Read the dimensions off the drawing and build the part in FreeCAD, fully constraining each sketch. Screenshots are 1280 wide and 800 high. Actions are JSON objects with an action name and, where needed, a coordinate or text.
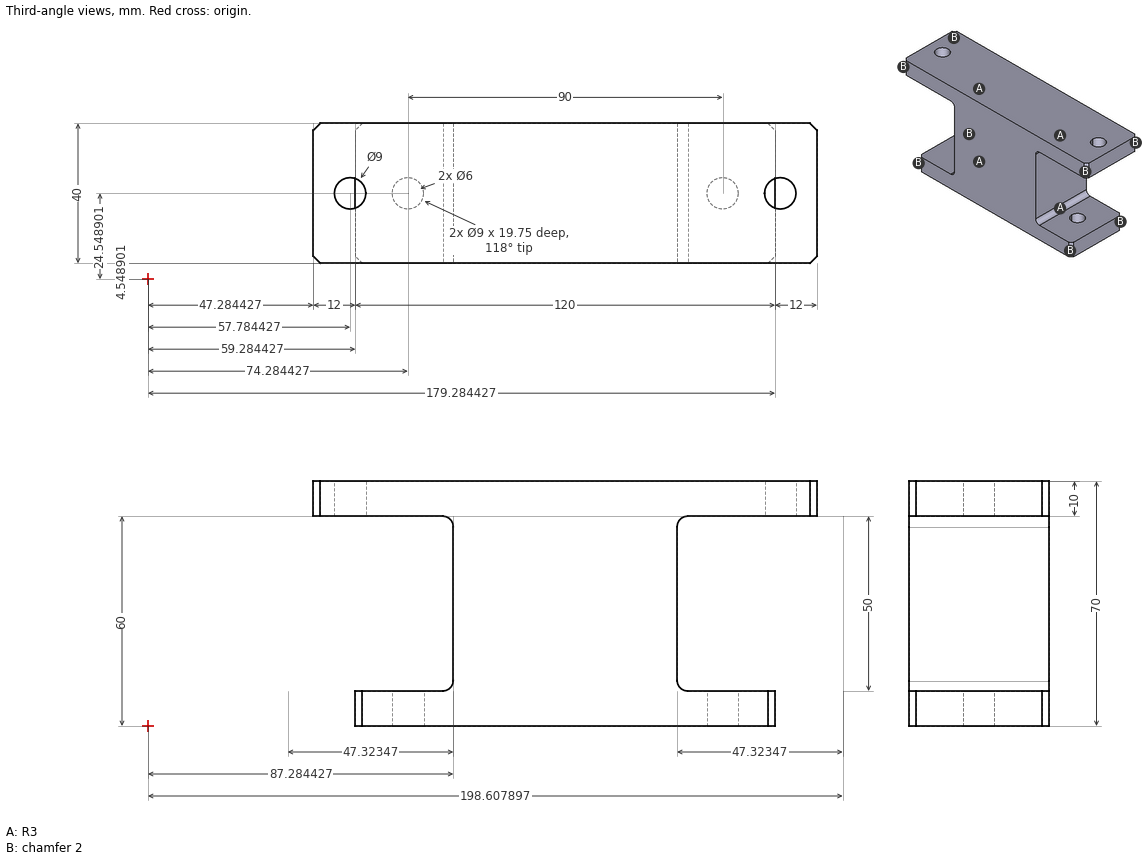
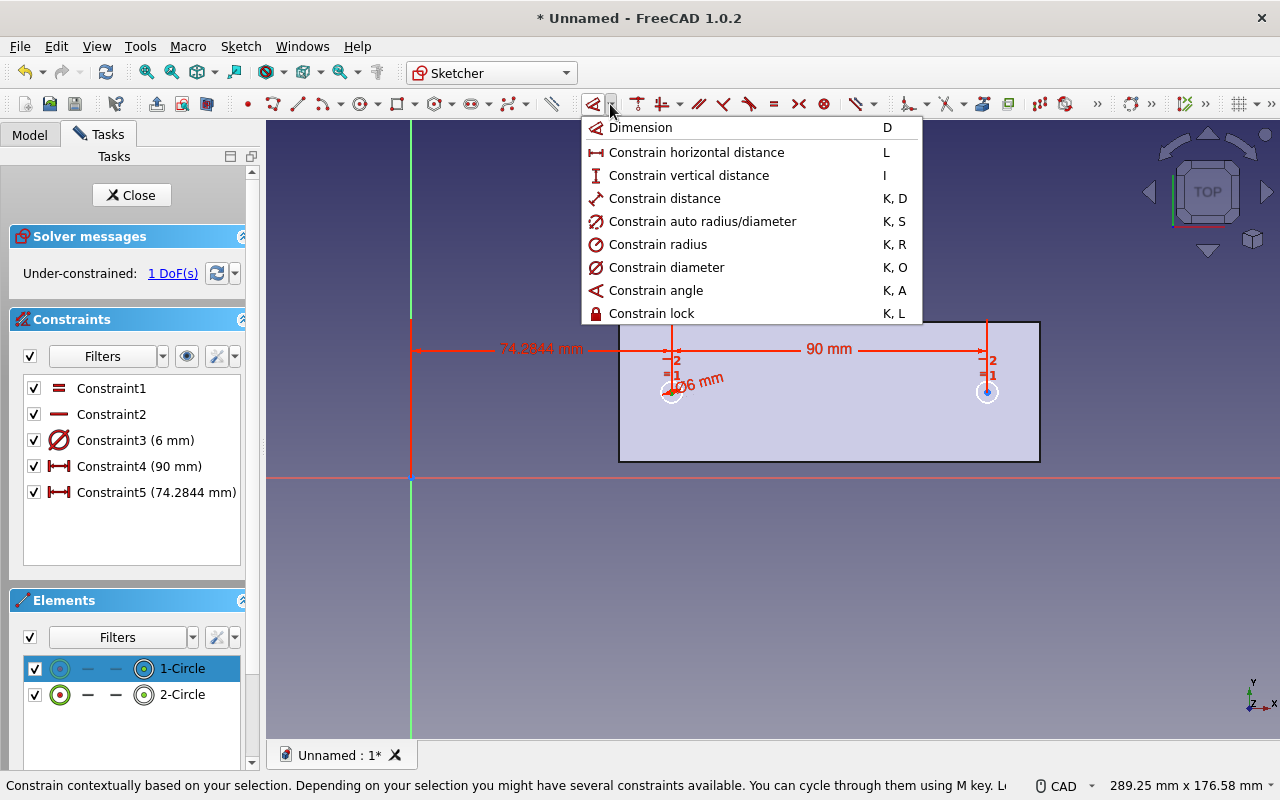
{"action": "left_click", "coordinate": [752, 176]}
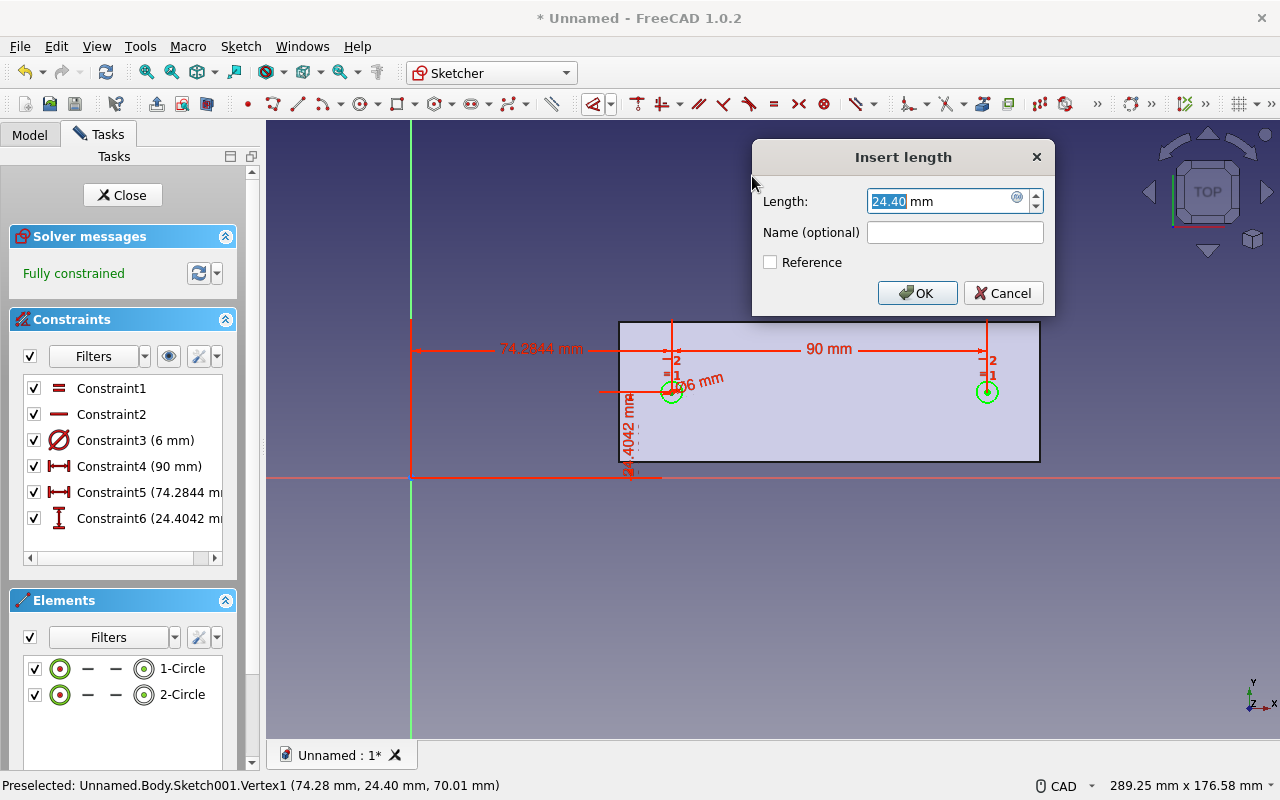
{"action": "type", "text": "24.548901"}
{"action": "key", "text": "Return"}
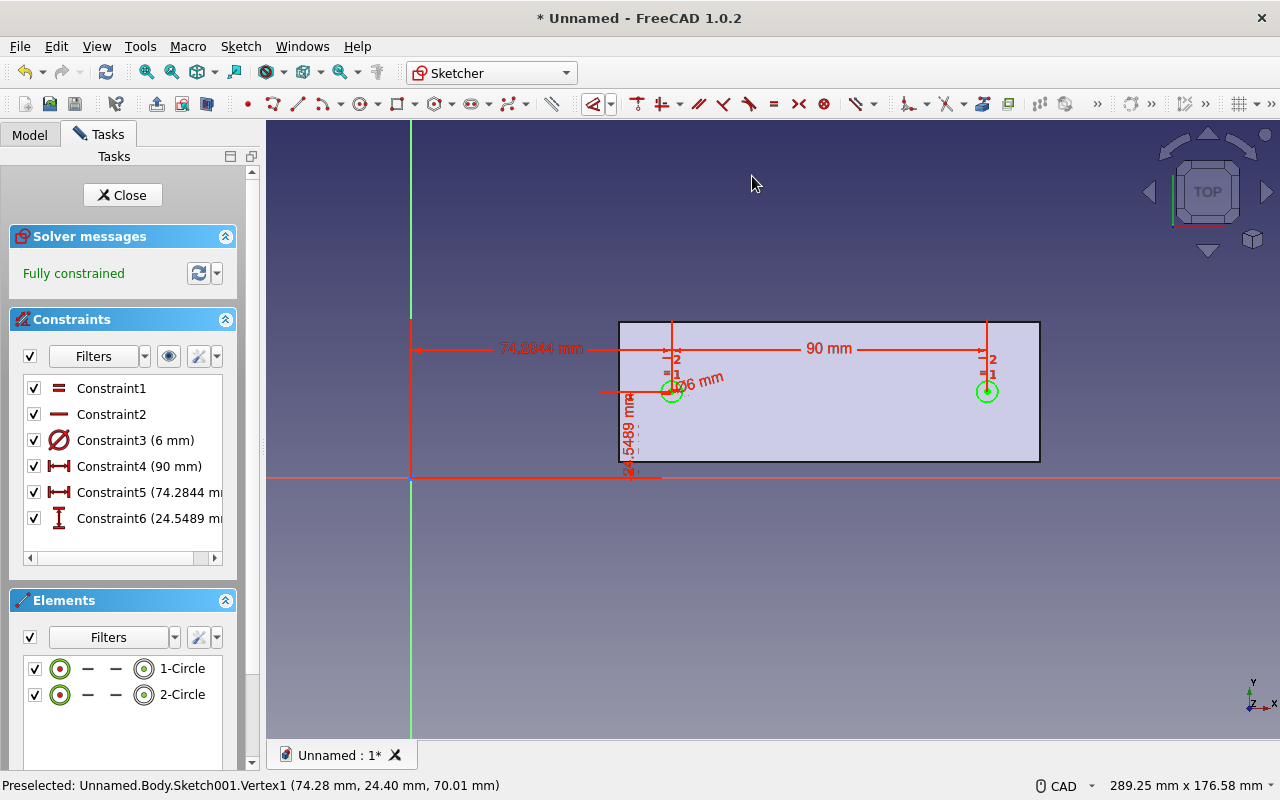
{"action": "left_click", "coordinate": [123, 195]}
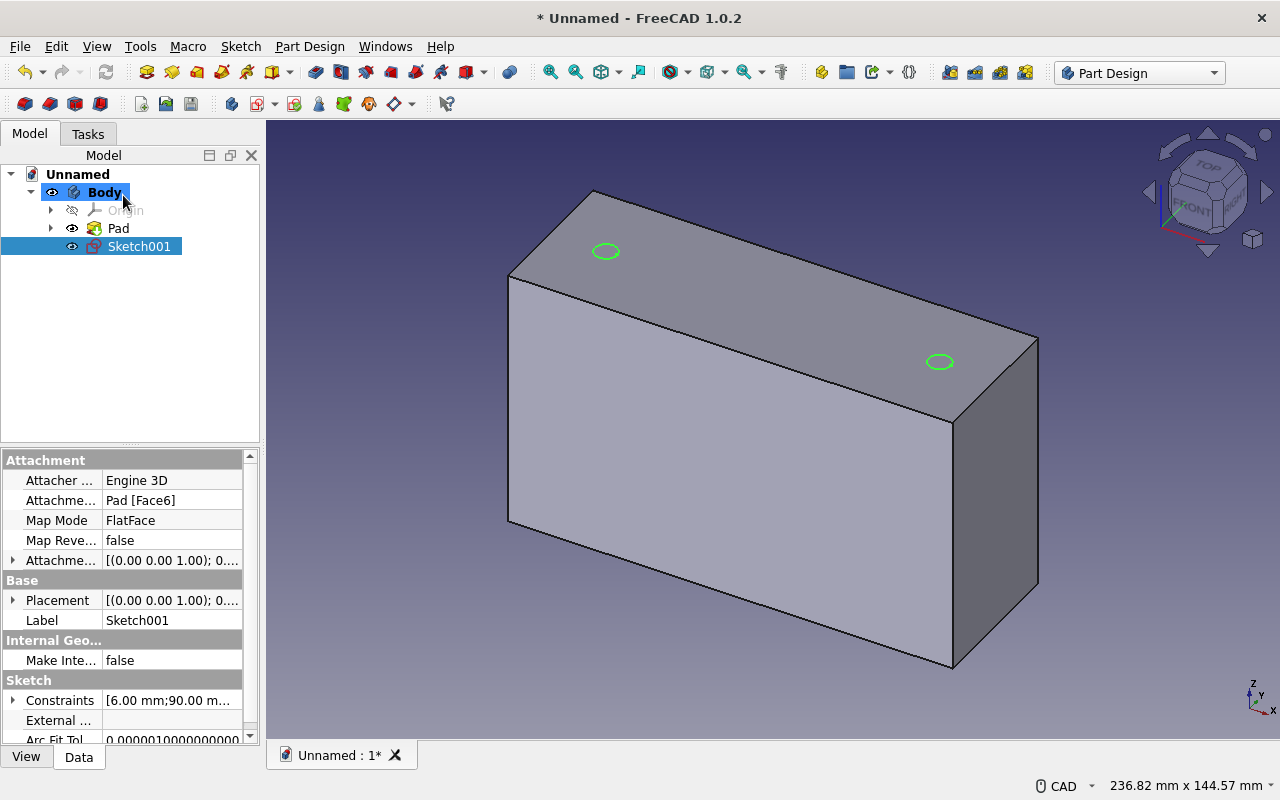
{"action": "left_click", "coordinate": [316, 72]}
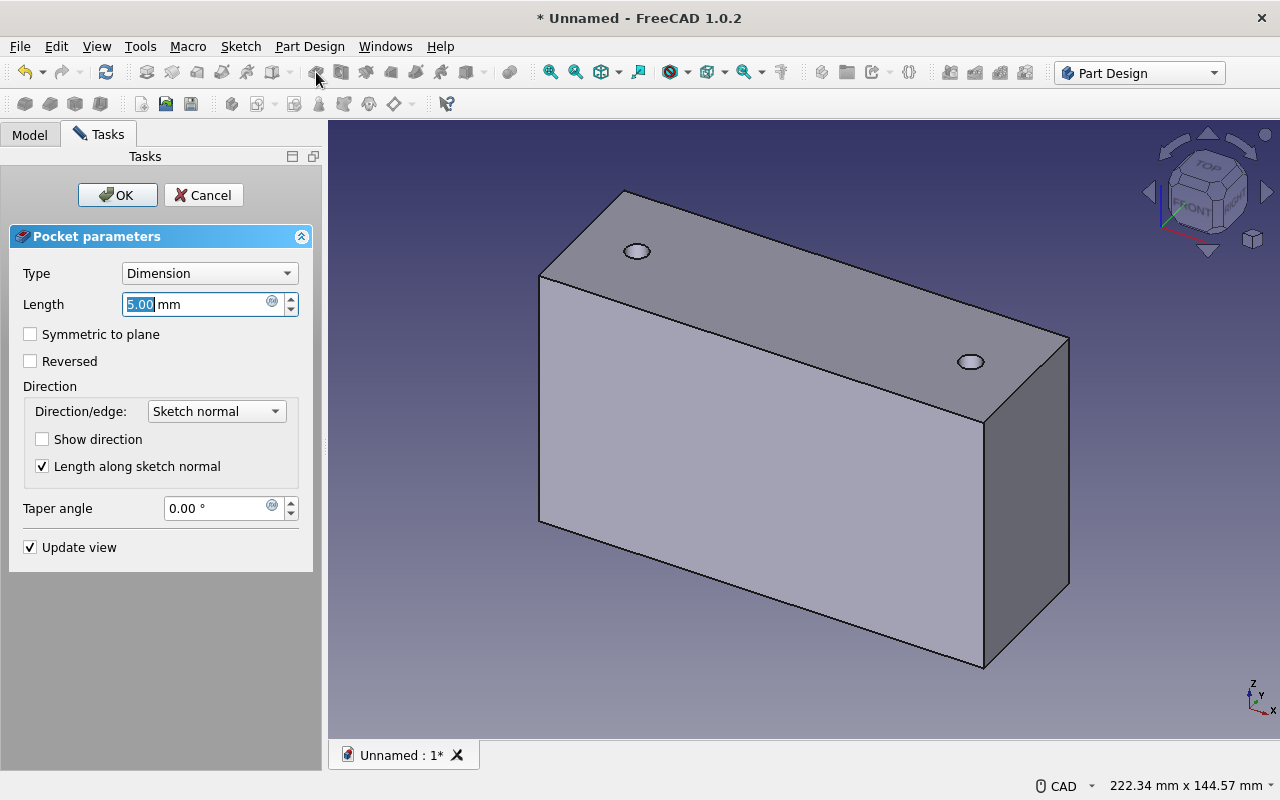
{"action": "left_click", "coordinate": [210, 274]}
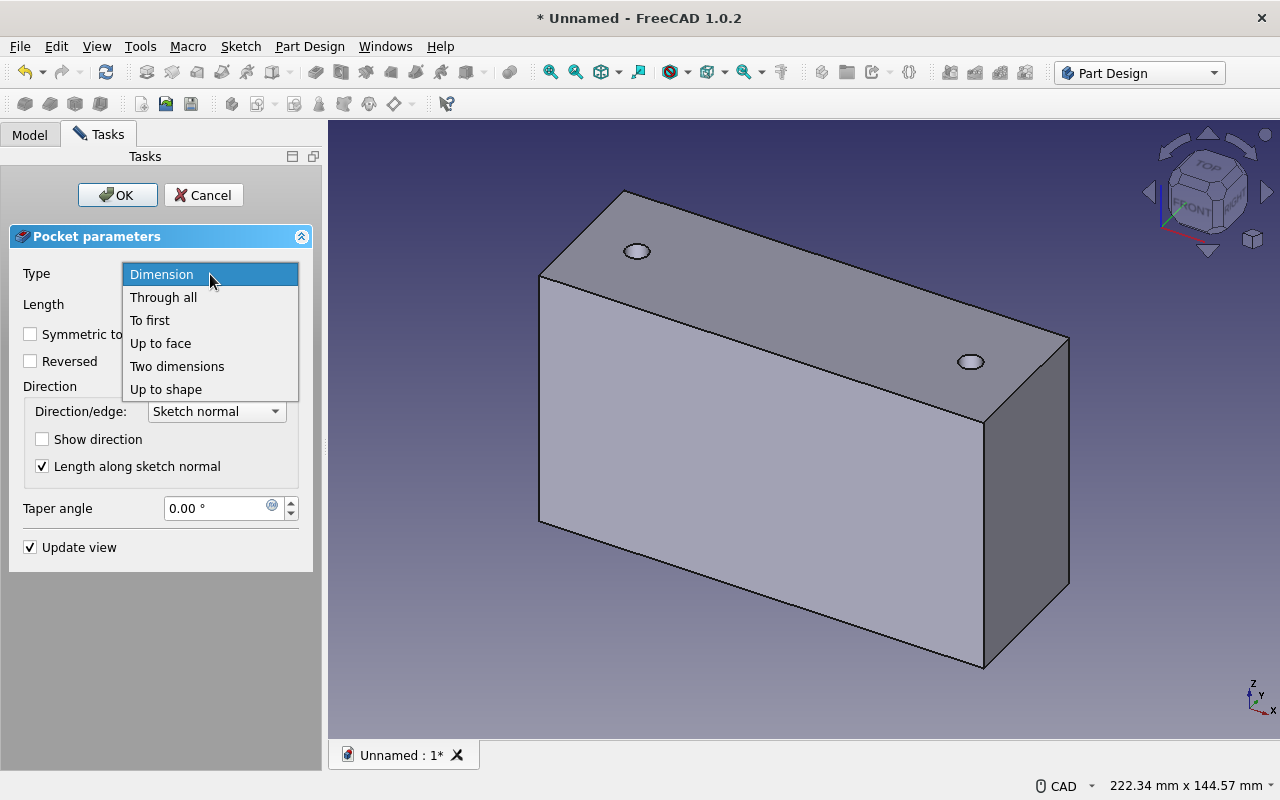
{"action": "left_click", "coordinate": [208, 298]}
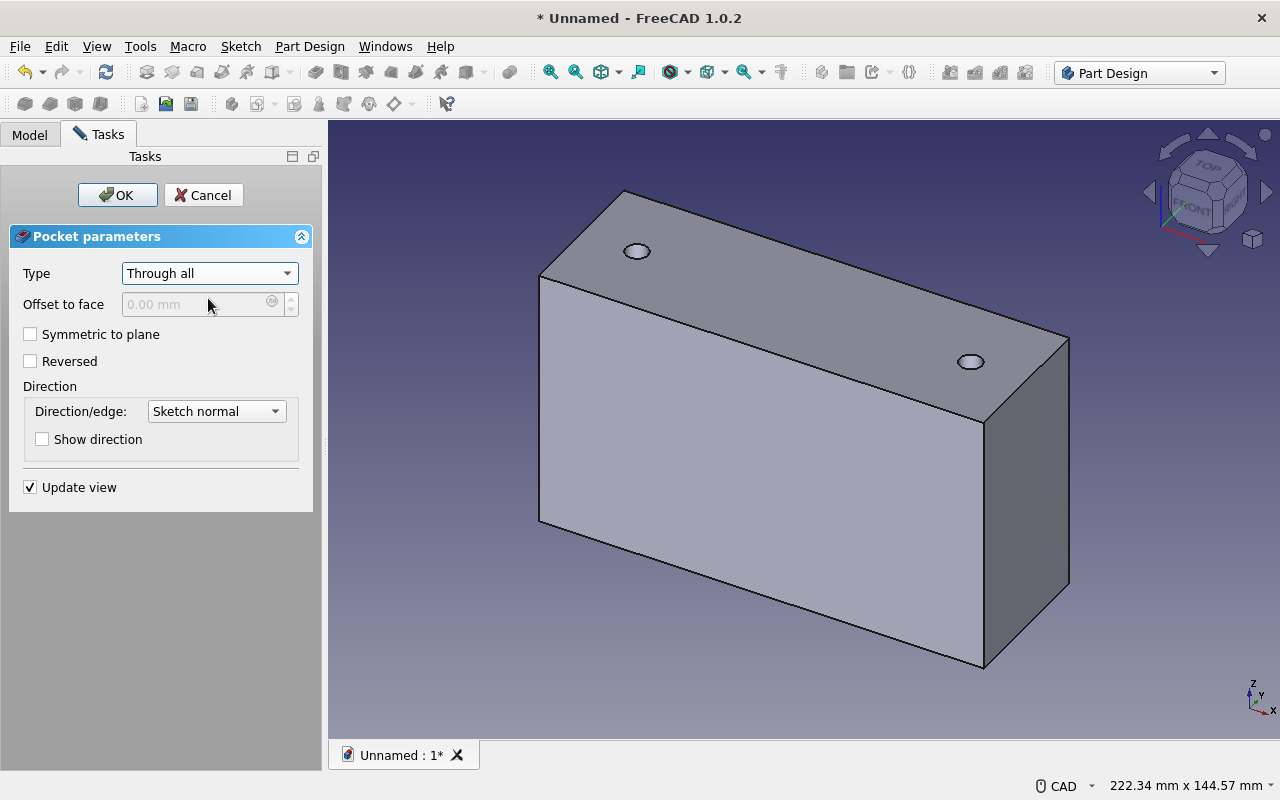
{"action": "left_click", "coordinate": [118, 195]}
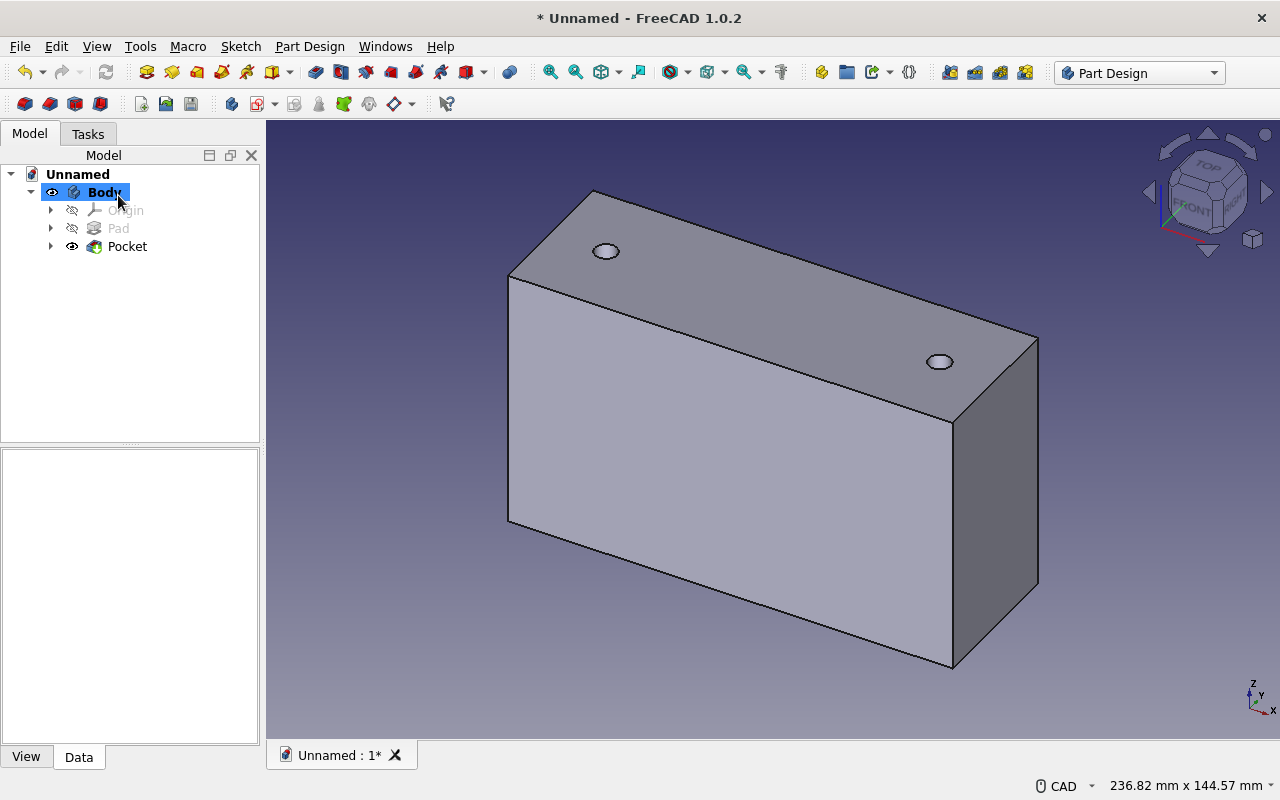
{"action": "key", "text": "4"}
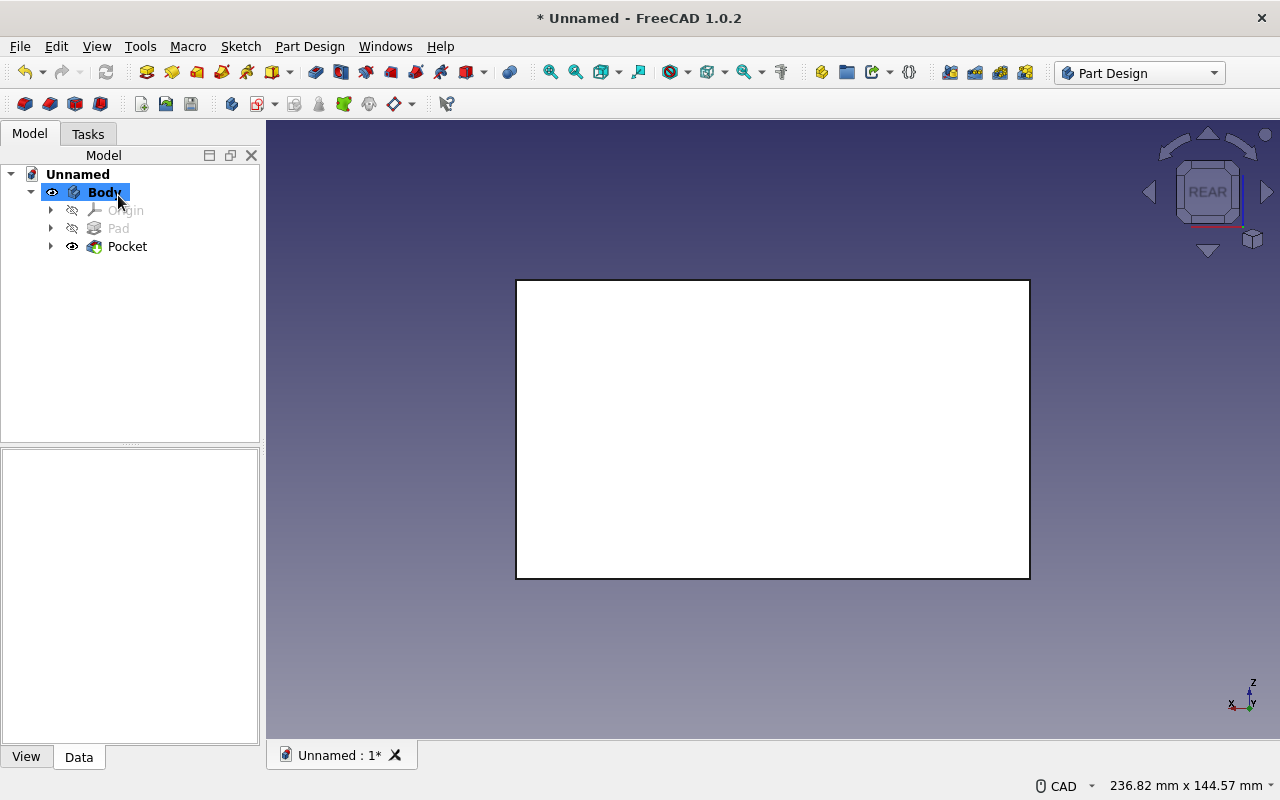
{"action": "left_click", "coordinate": [700, 428]}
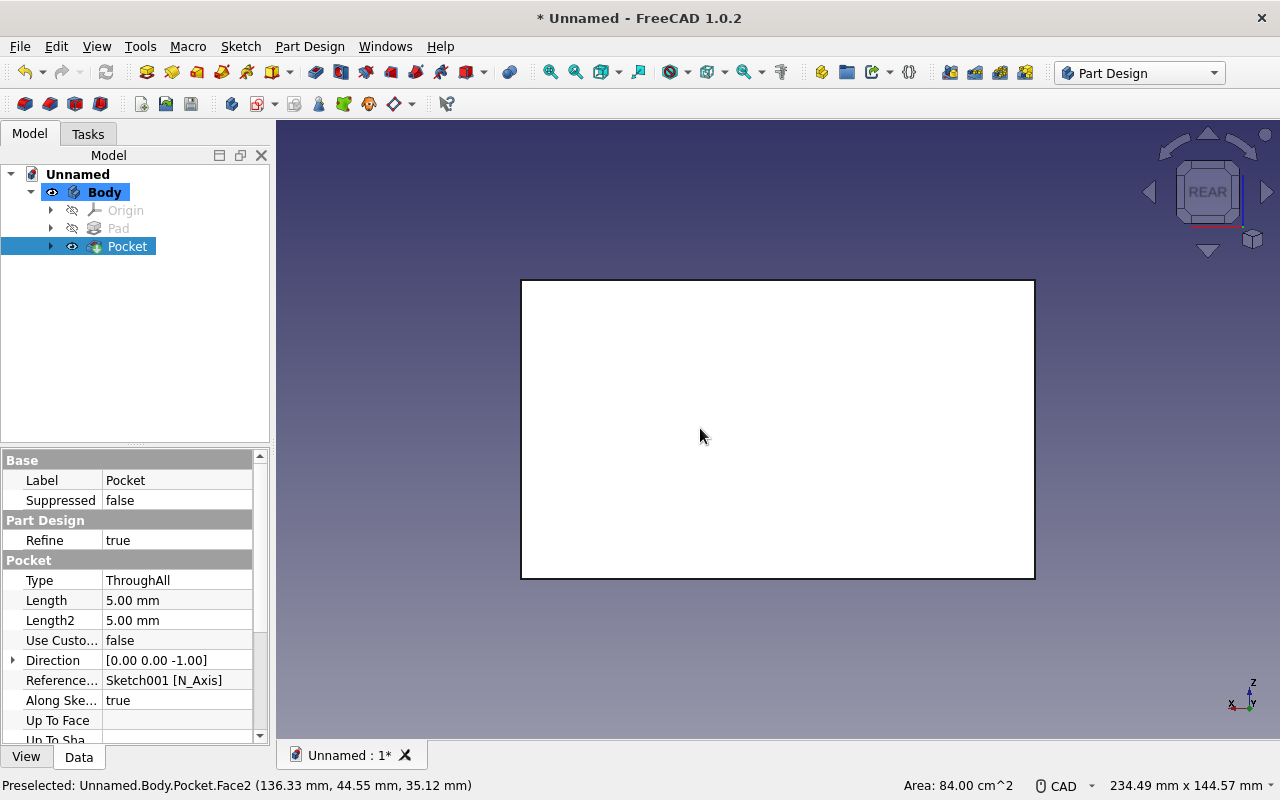
{"action": "left_click", "coordinate": [256, 104]}